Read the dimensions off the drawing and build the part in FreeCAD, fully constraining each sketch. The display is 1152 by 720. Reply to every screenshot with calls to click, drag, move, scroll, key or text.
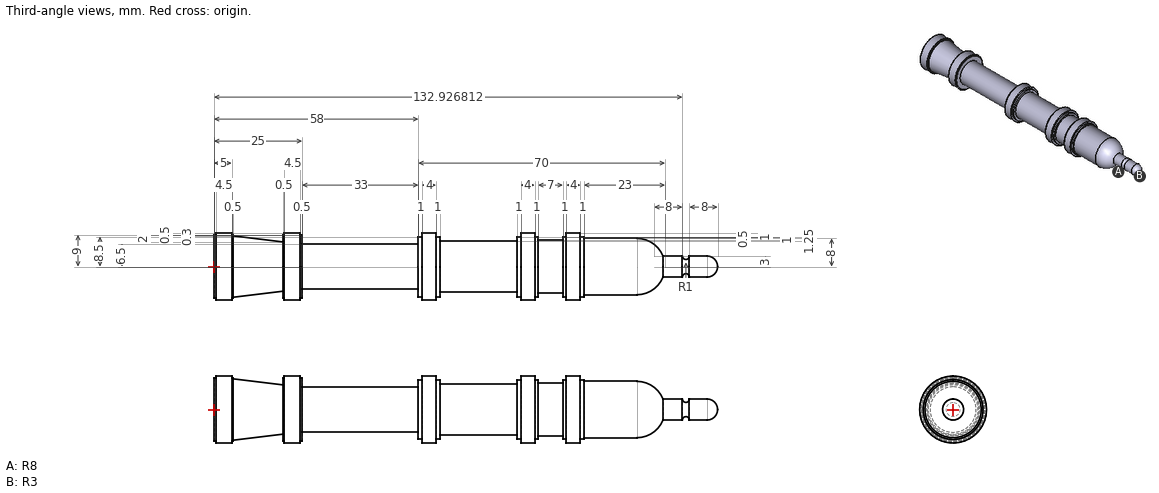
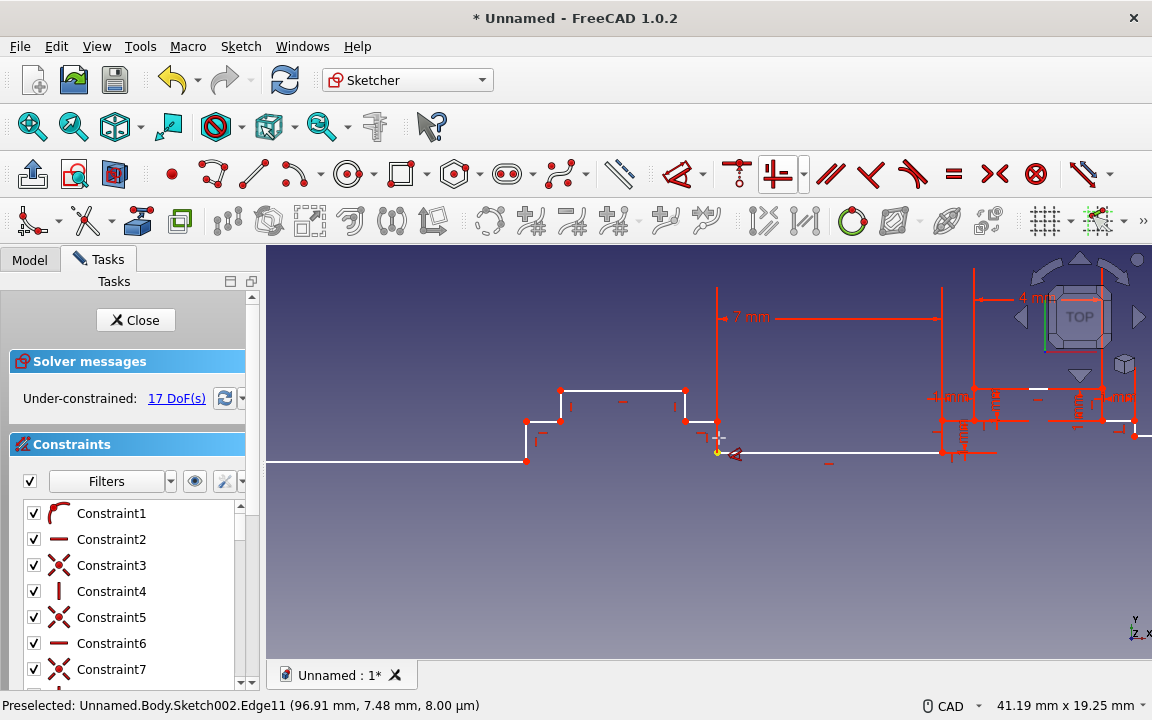
click(716, 437)
click(750, 437)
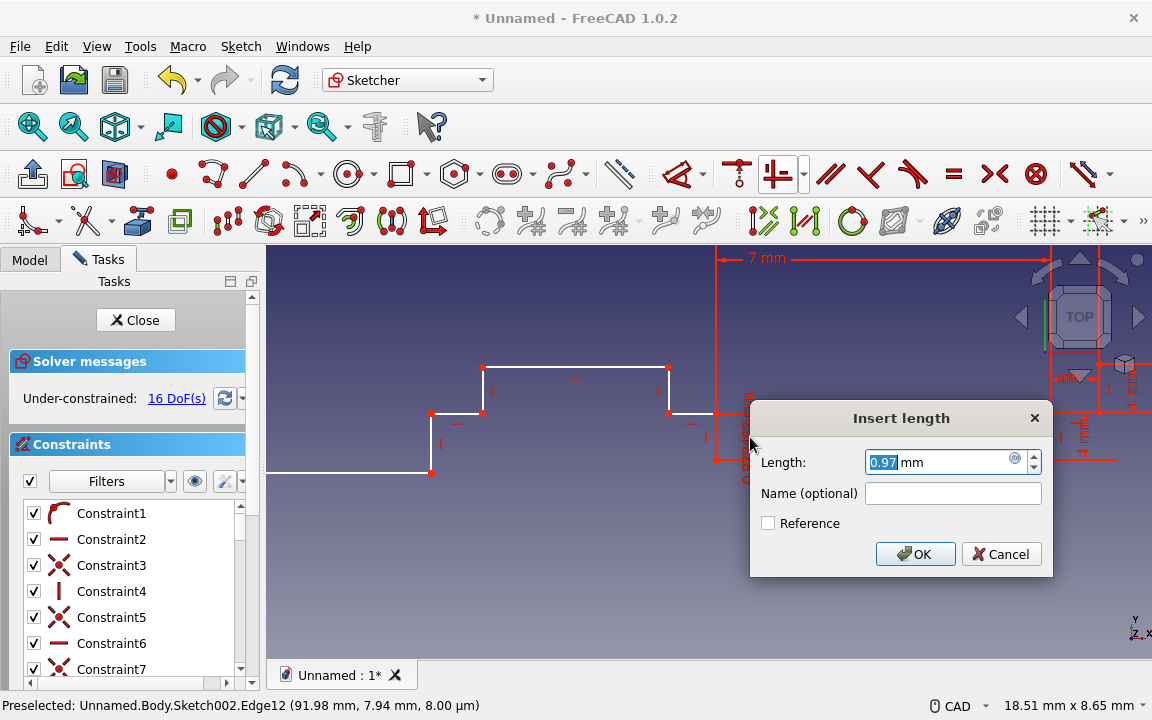
text(1)
key(Return)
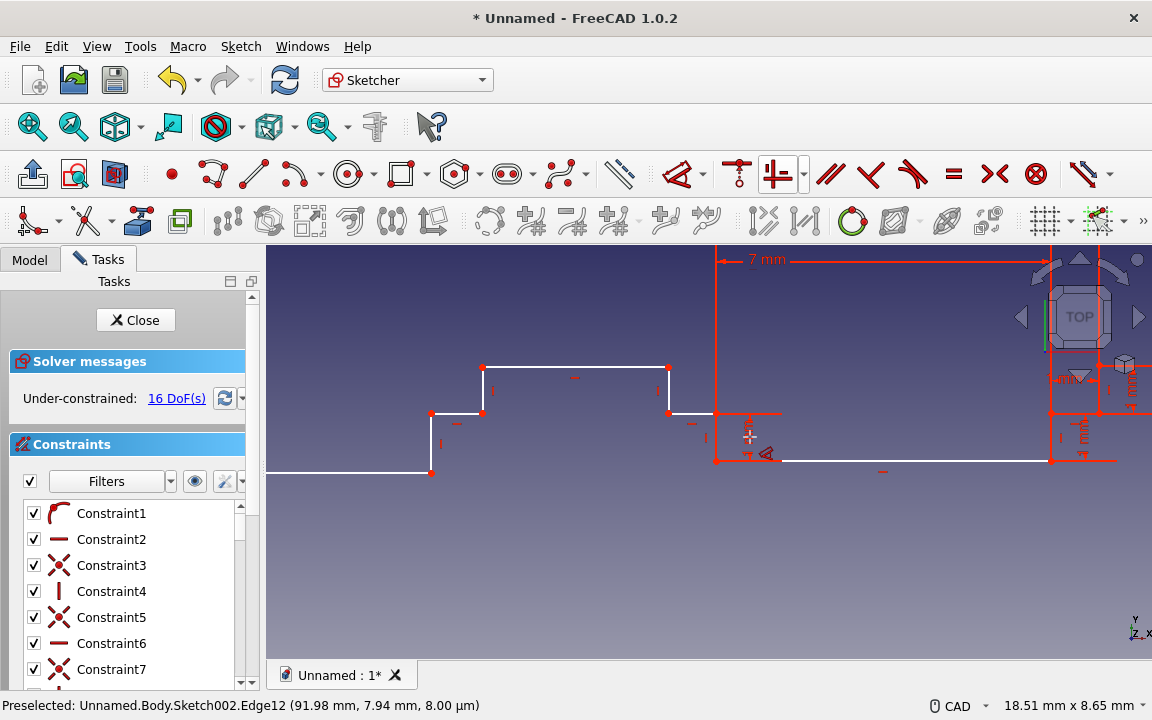
click(702, 414)
click(693, 380)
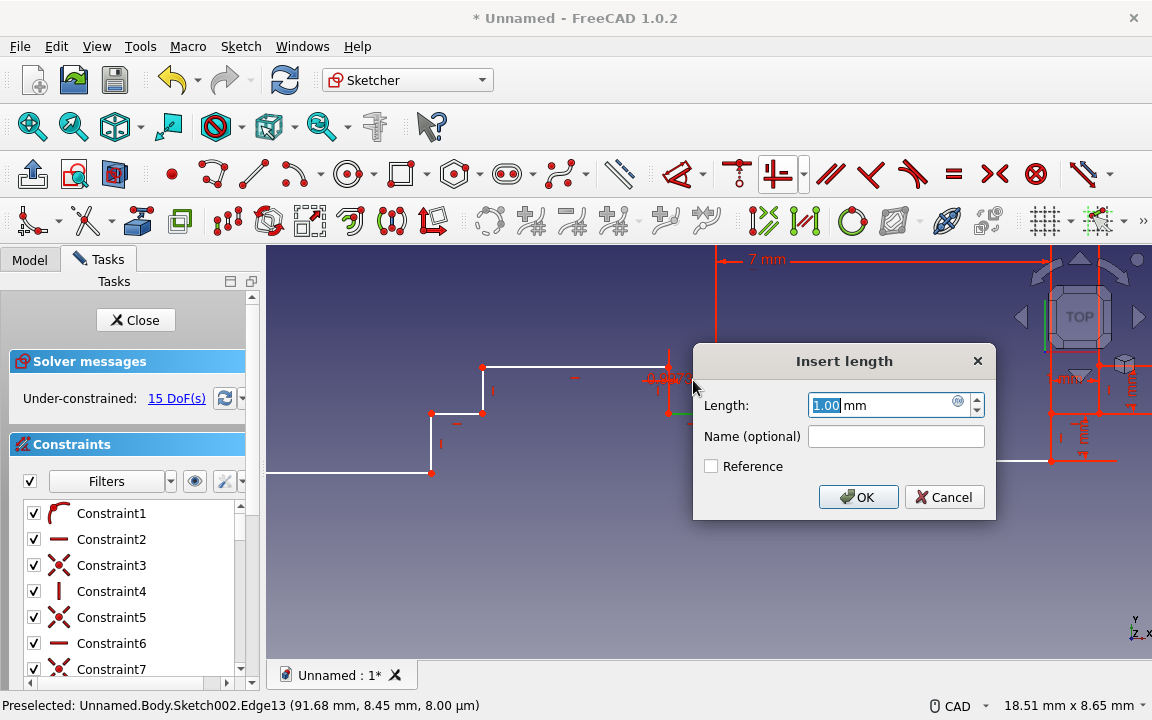
text(1)
key(Return)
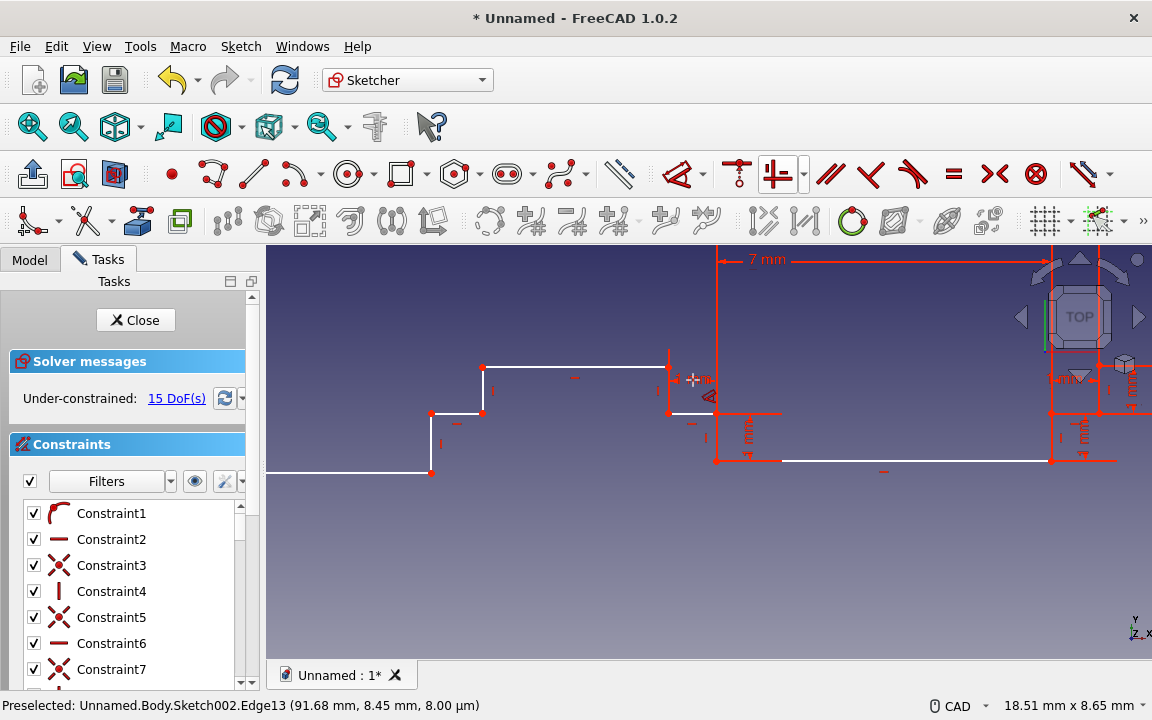
click(669, 400)
click(635, 401)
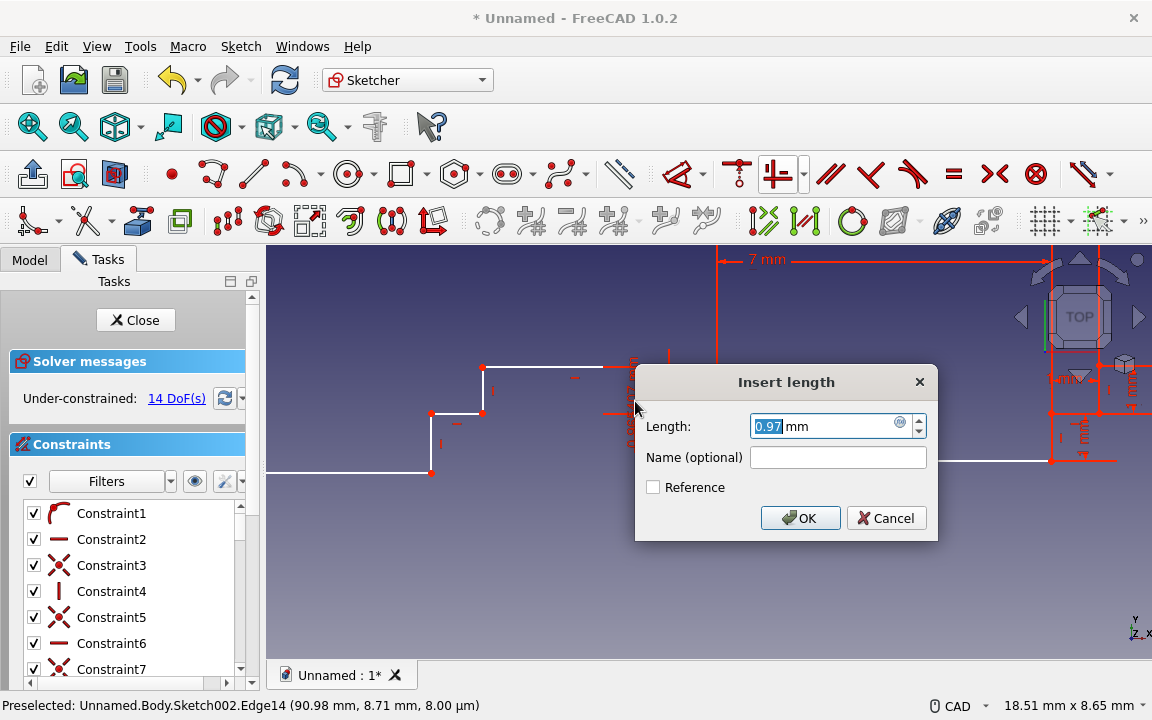
text(1)
key(Return)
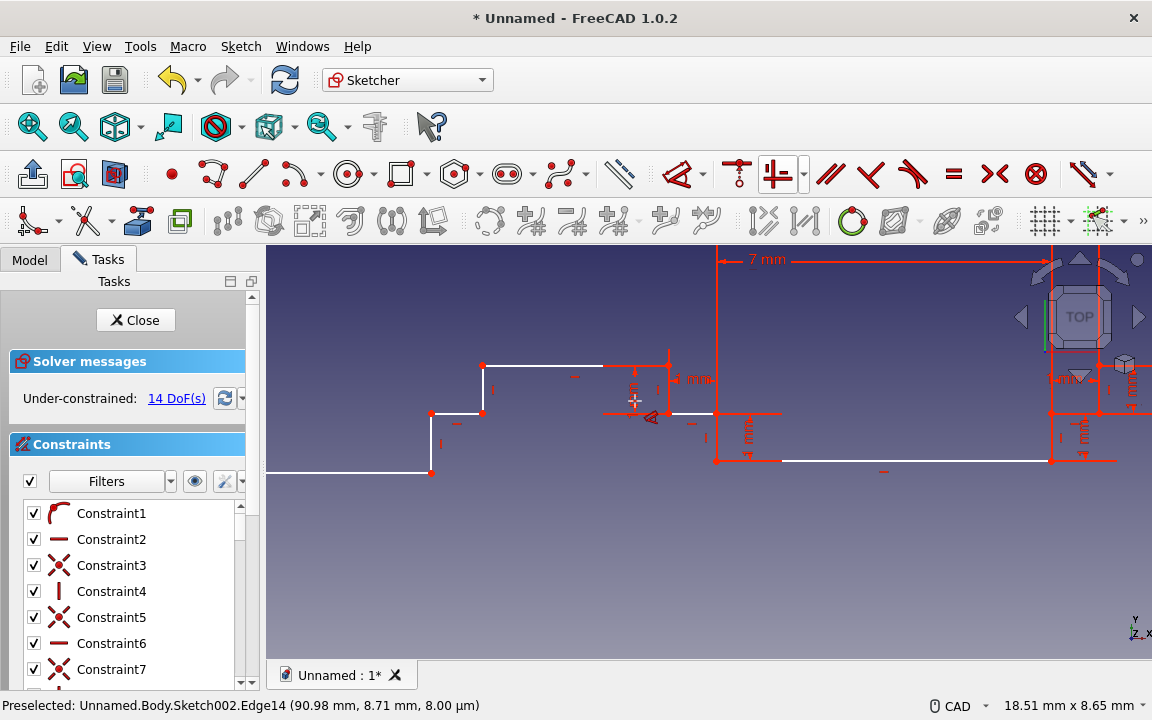
scroll(742, 441, down, 13)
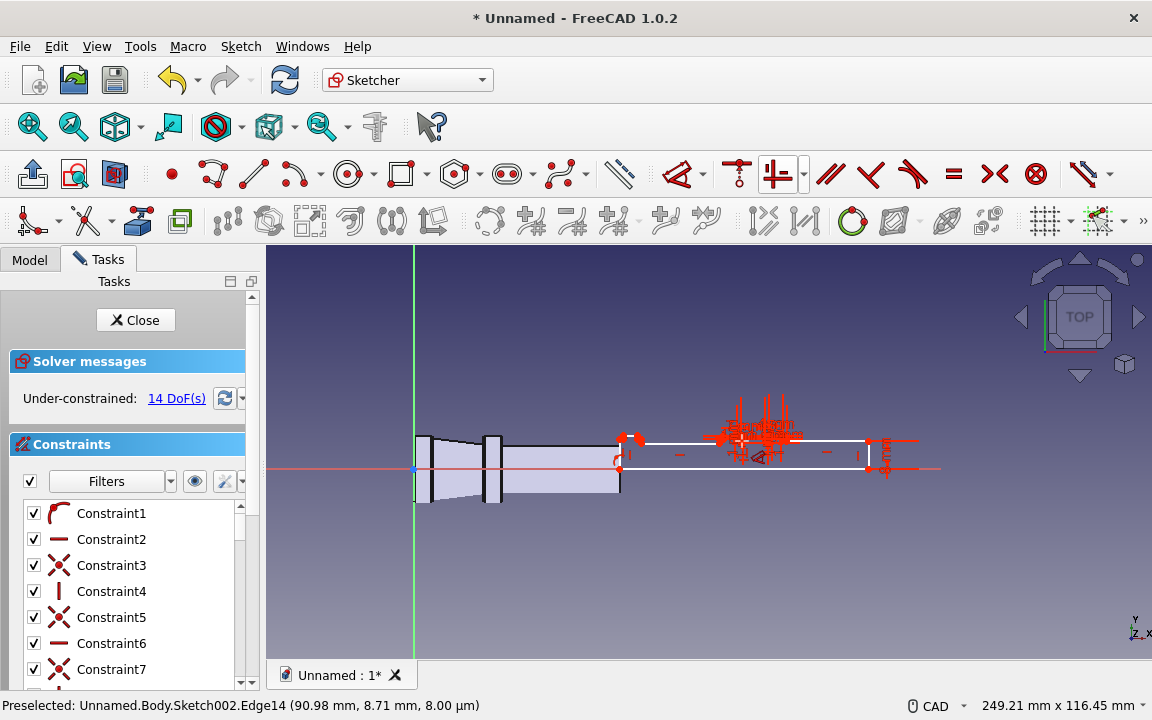
scroll(733, 436, up, 7)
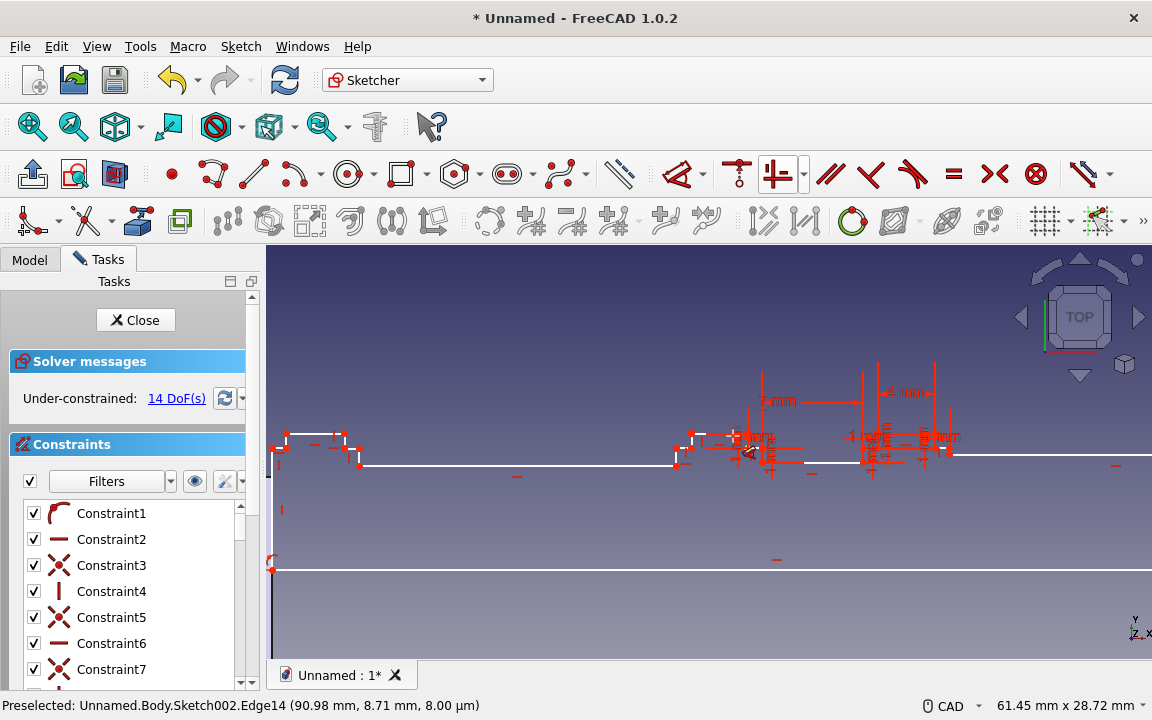
click(731, 434)
click(700, 400)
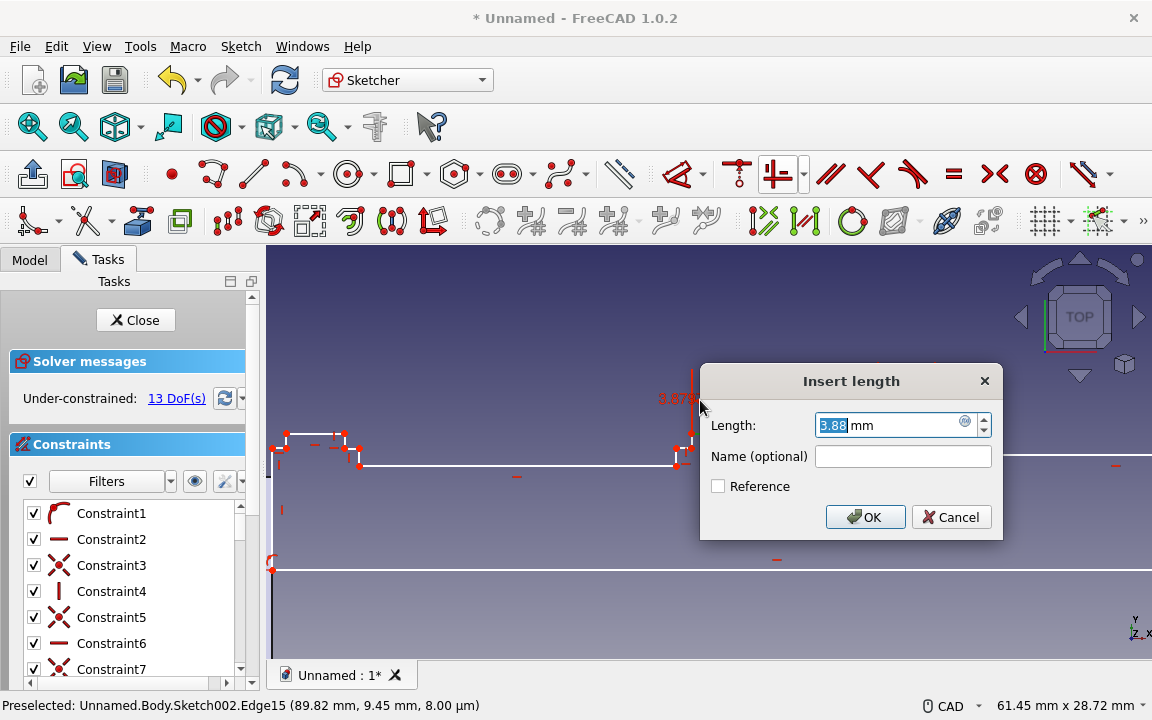
text(4)
key(Return)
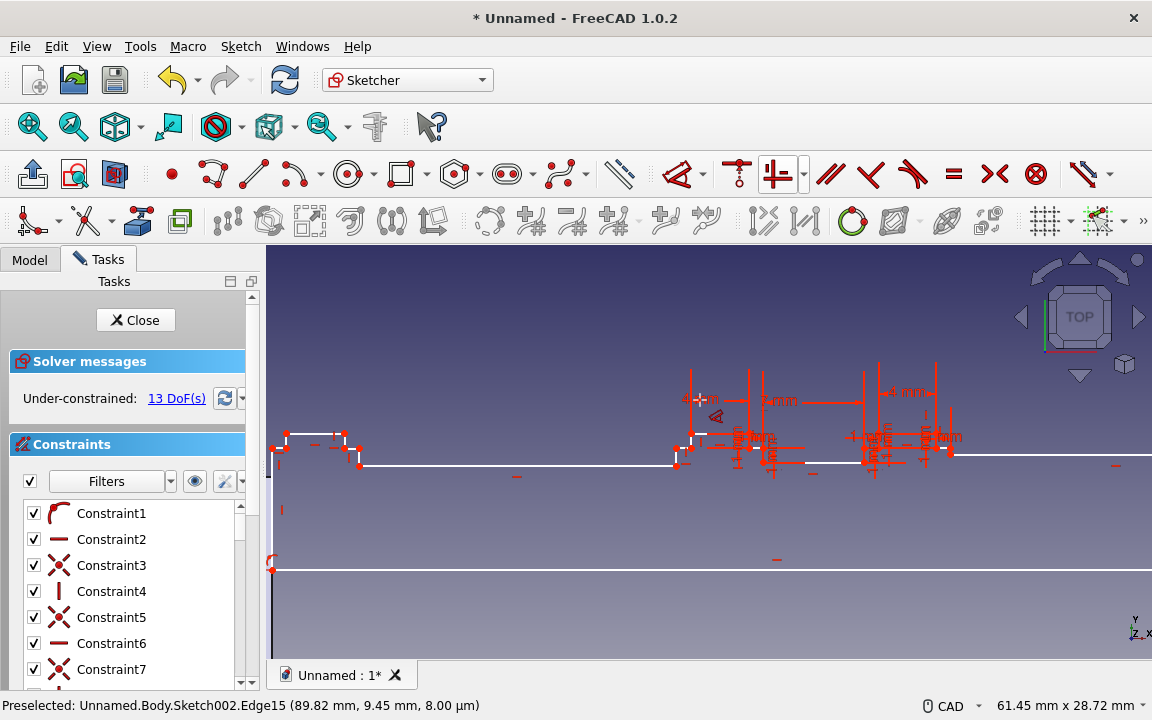
scroll(691, 441, up, 6)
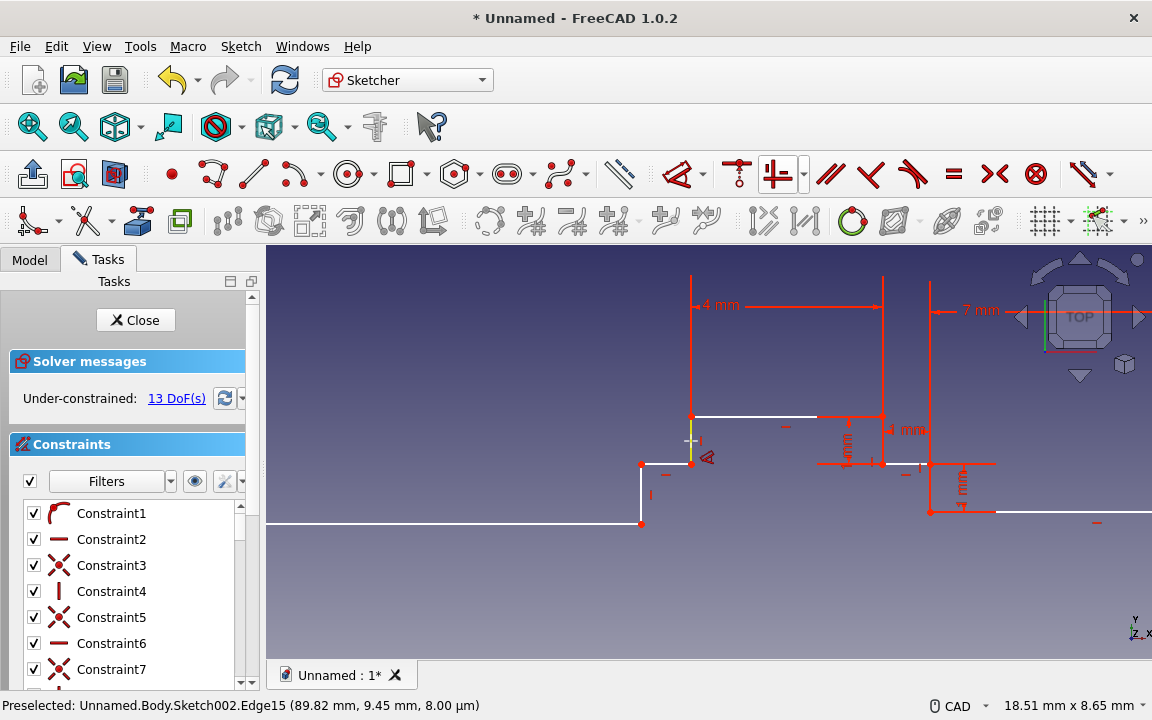
click(691, 440)
click(725, 440)